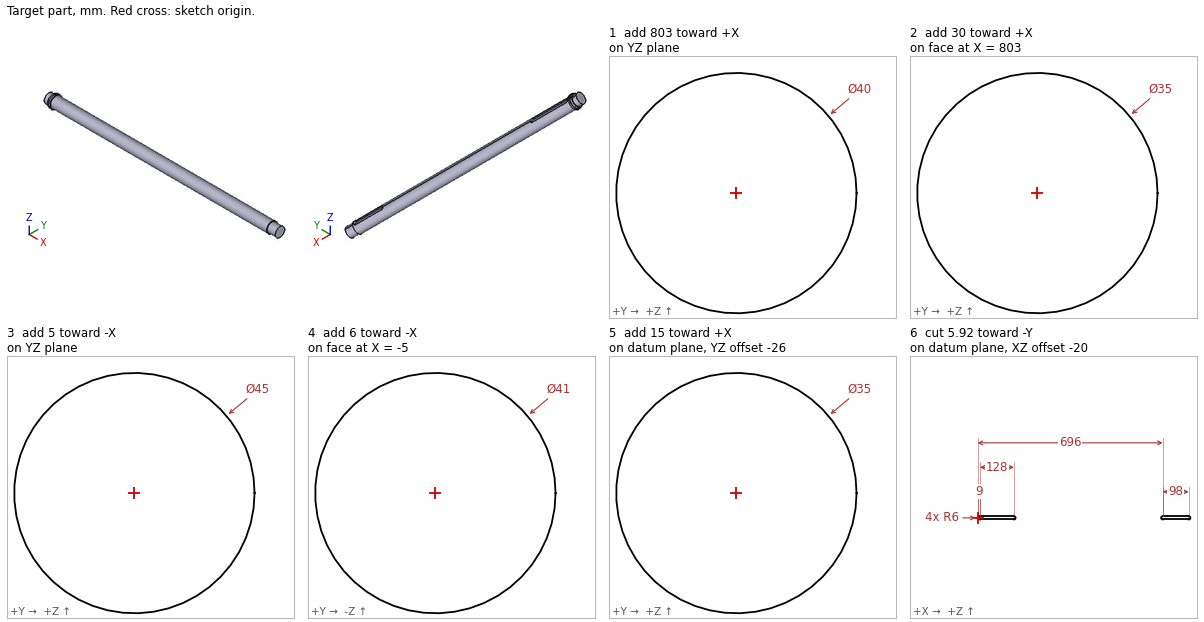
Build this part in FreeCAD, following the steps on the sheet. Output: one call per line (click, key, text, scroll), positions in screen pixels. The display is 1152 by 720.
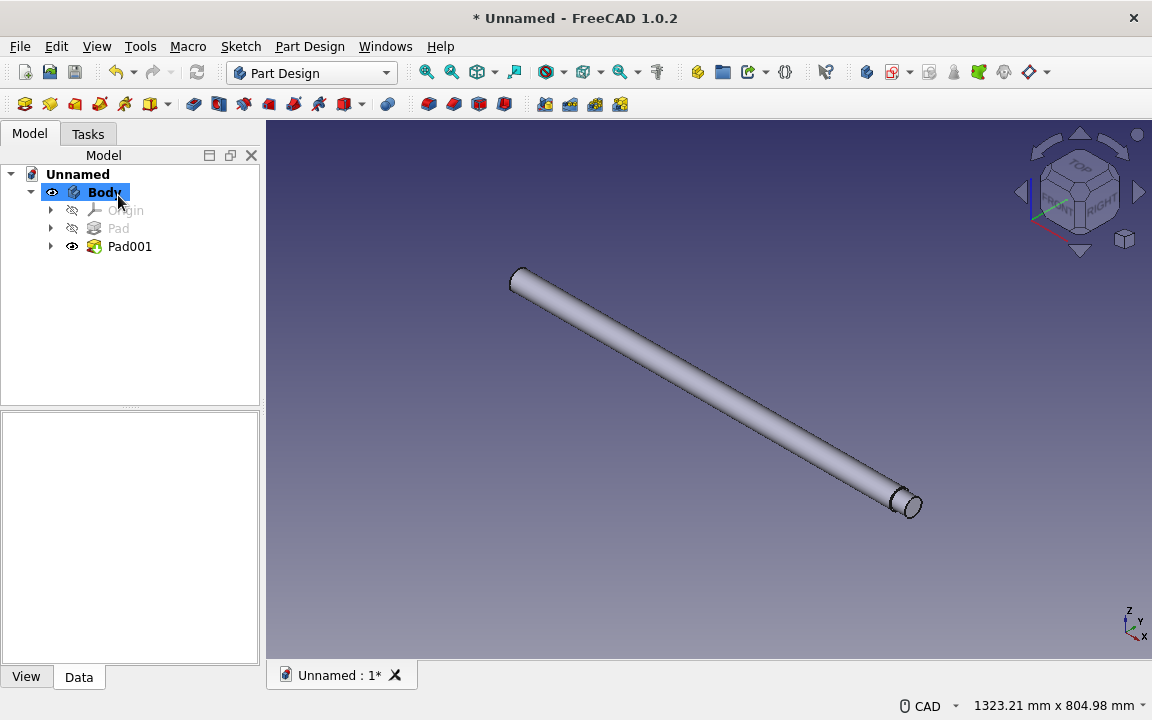
click(892, 72)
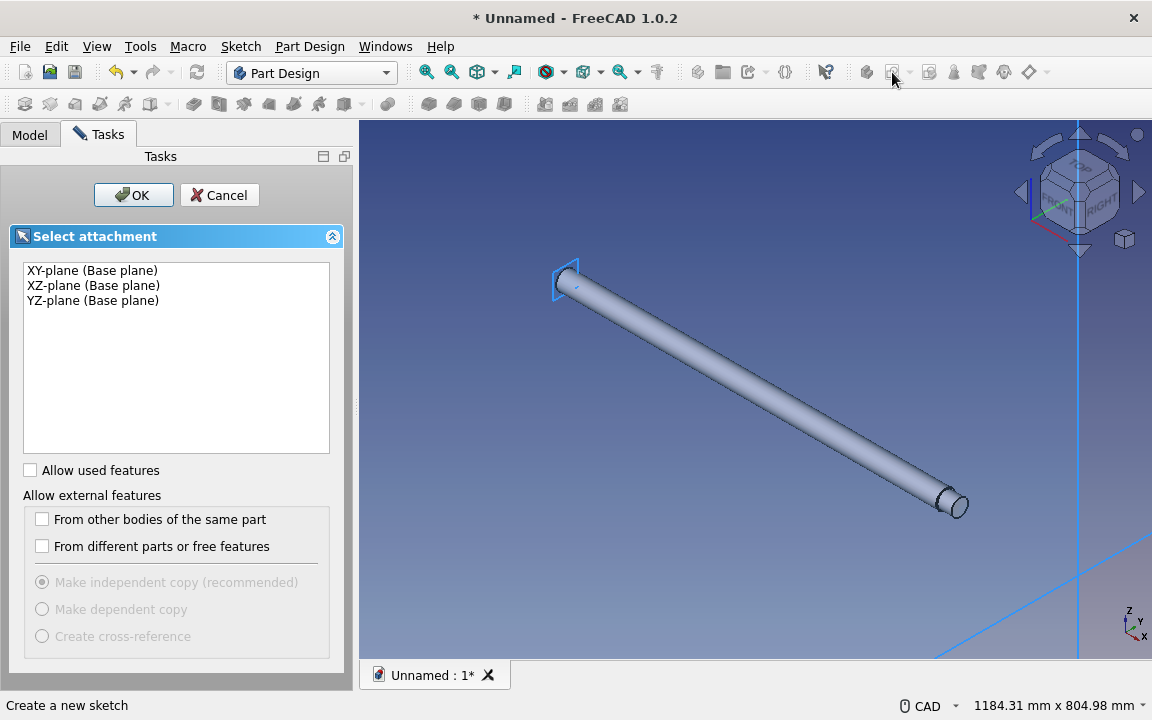
click(84, 300)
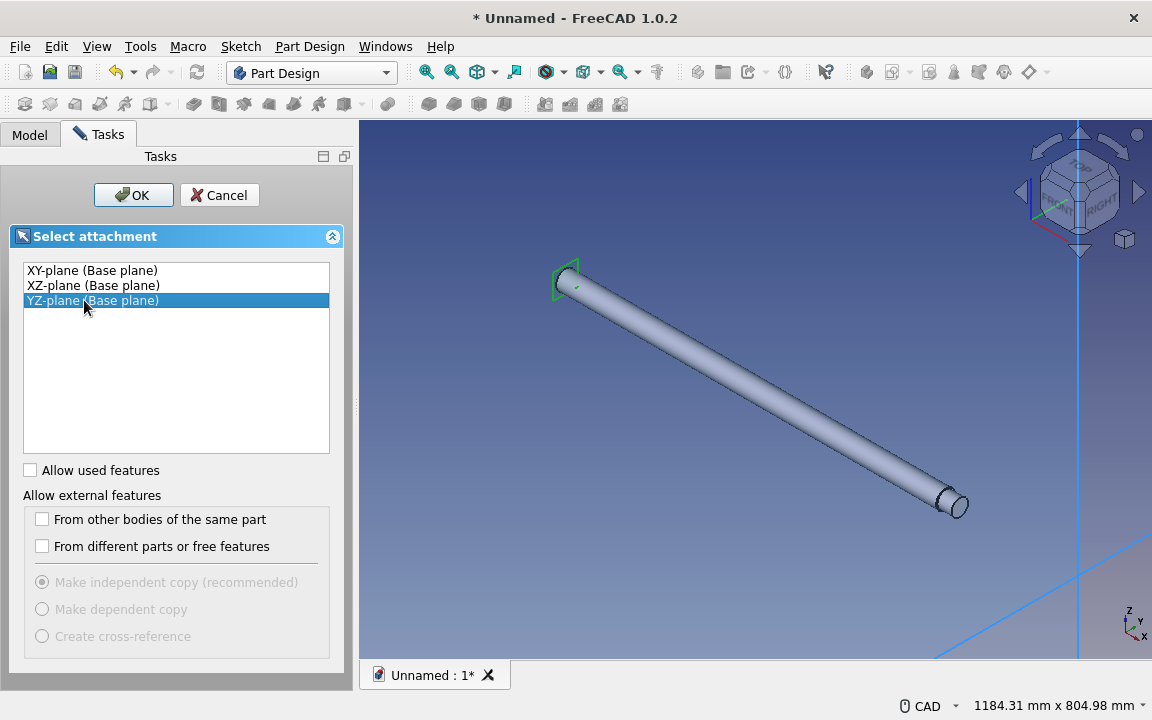
click(134, 195)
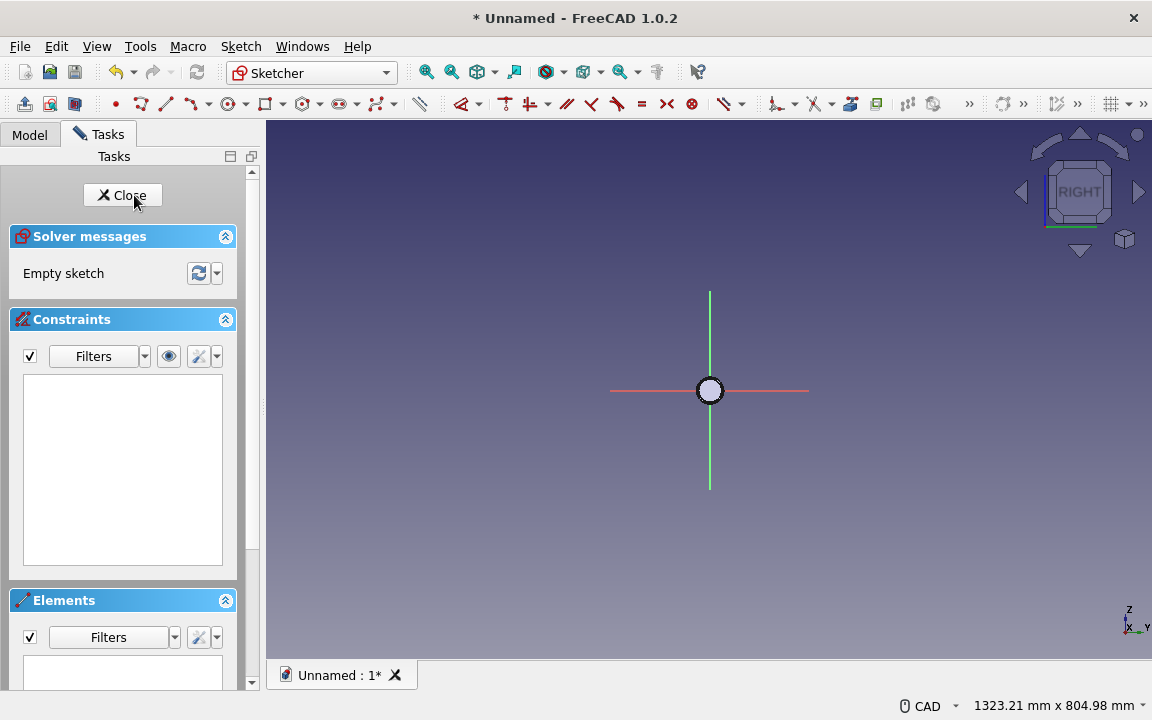
click(75, 104)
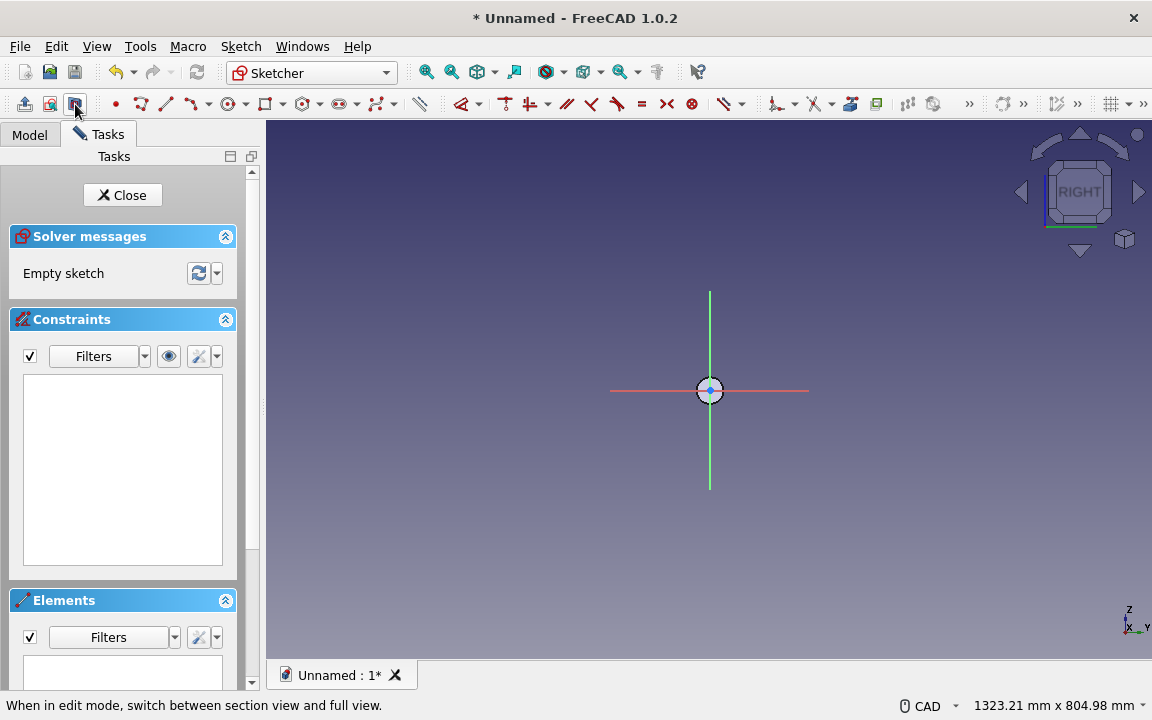
scroll(717, 391, up, 12)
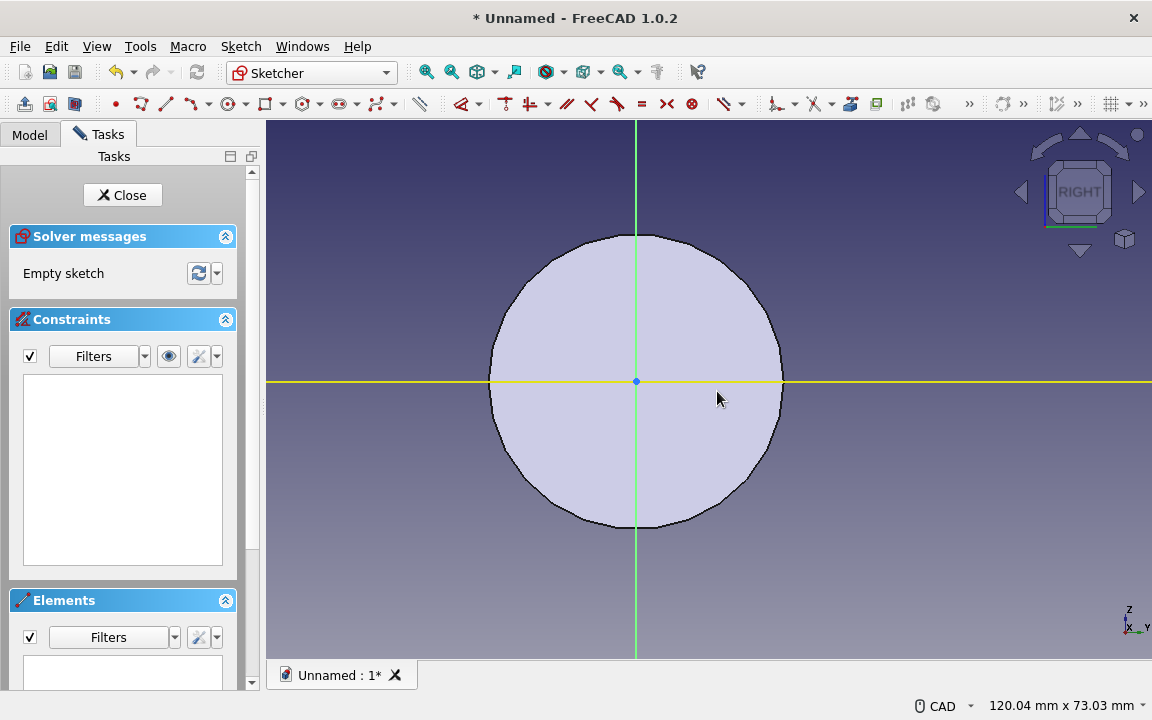
click(228, 104)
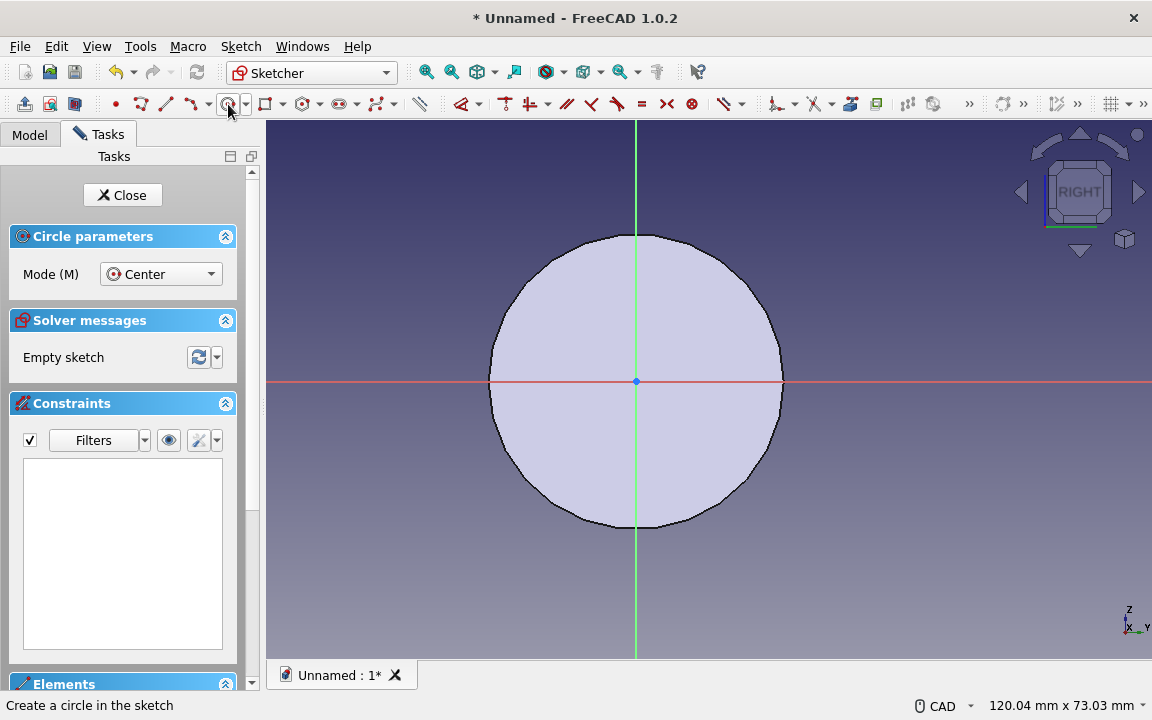
click(636, 382)
move(754, 264)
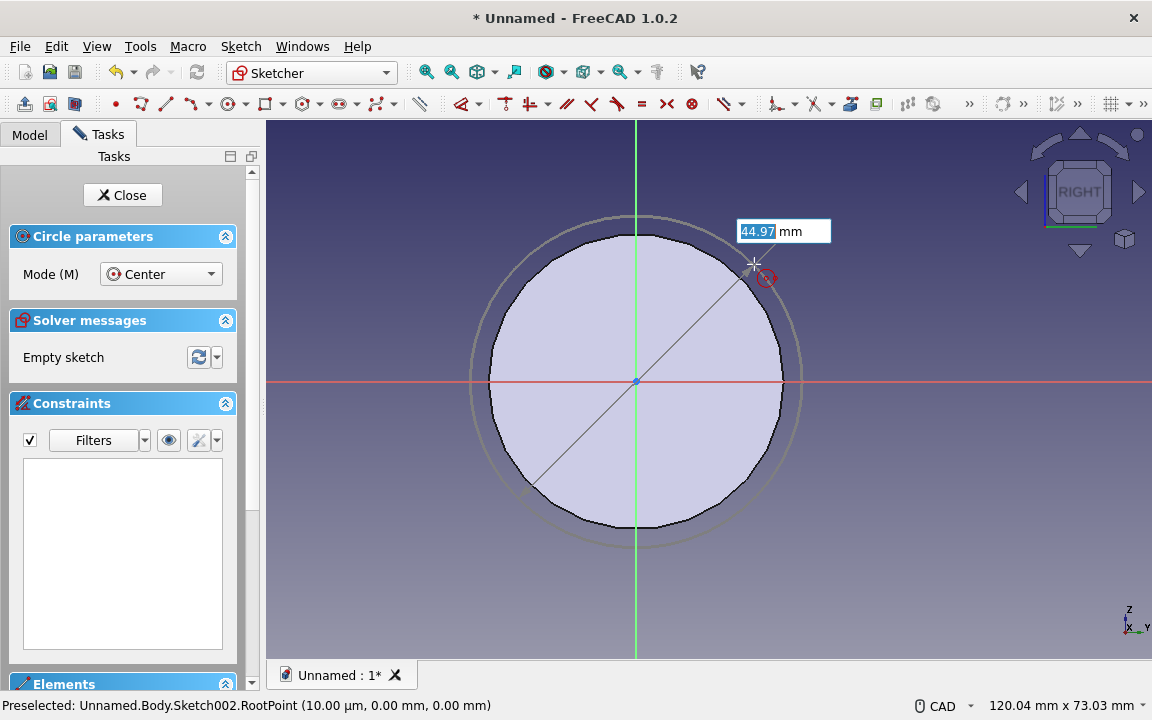
text(45)
key(Return)
key(Escape)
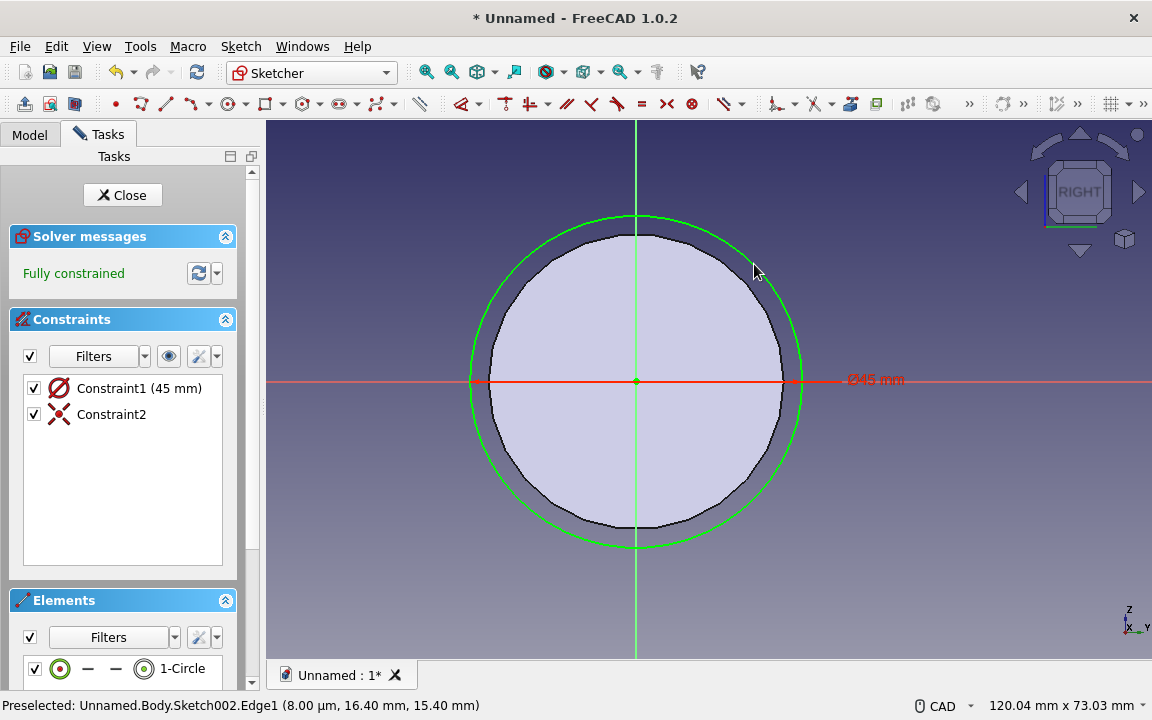
click(123, 195)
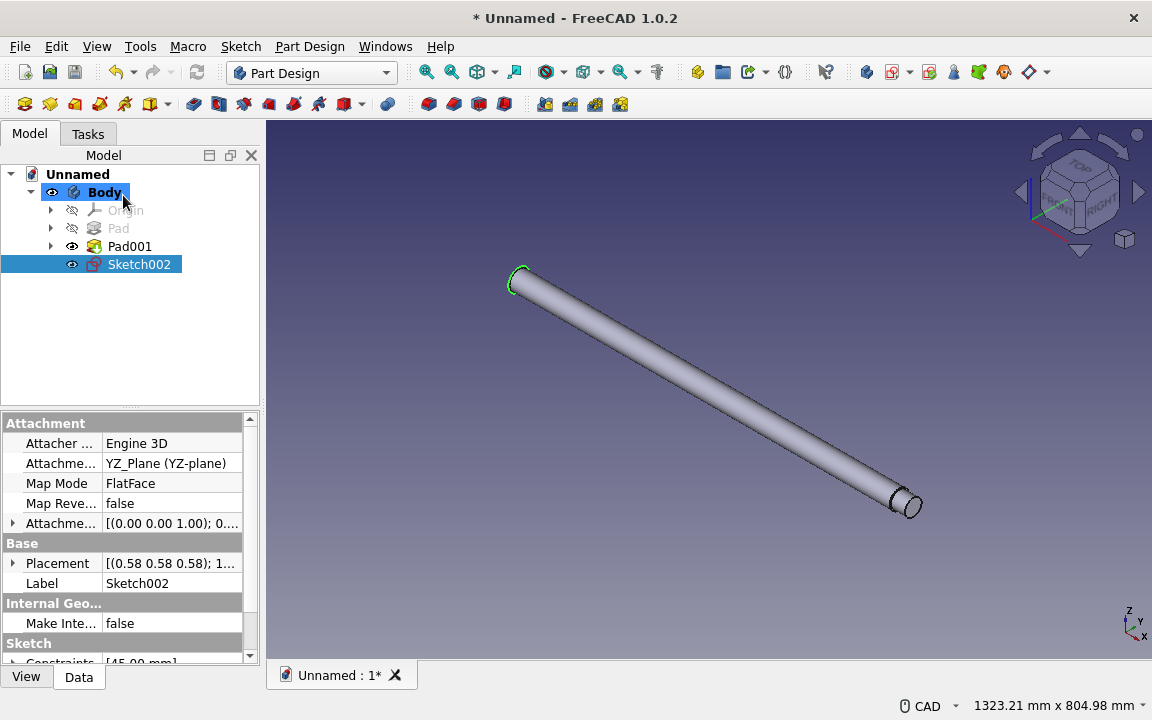
click(25, 104)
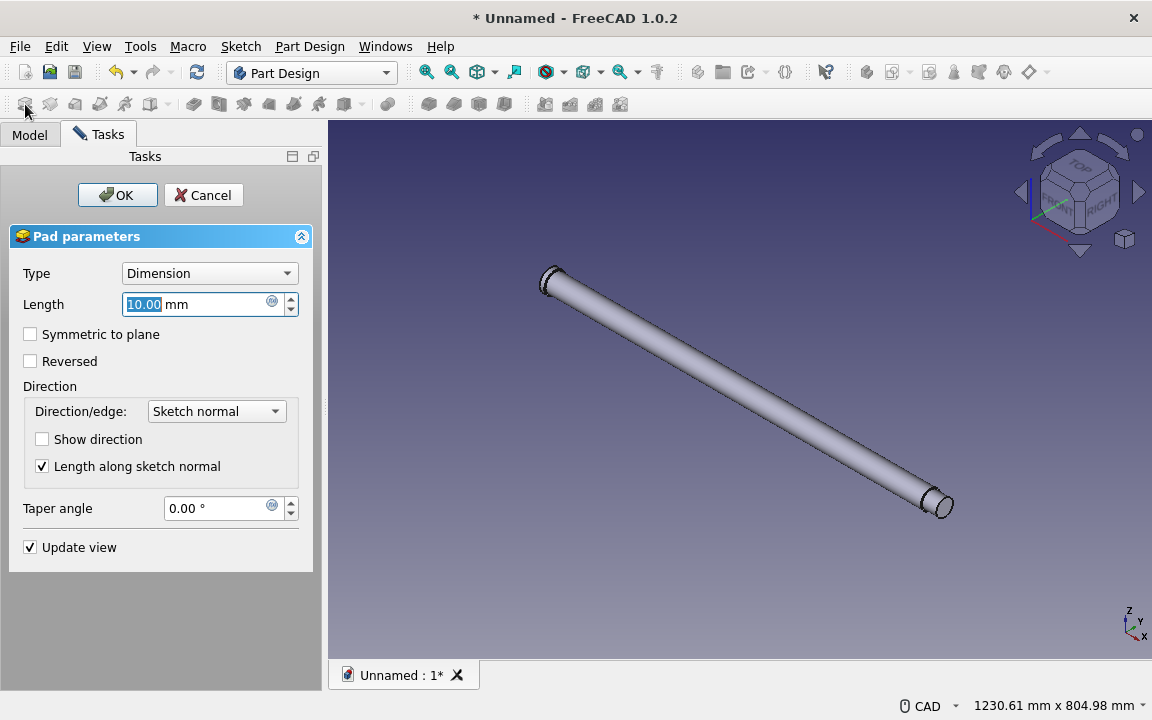
text(5)
key(Tab)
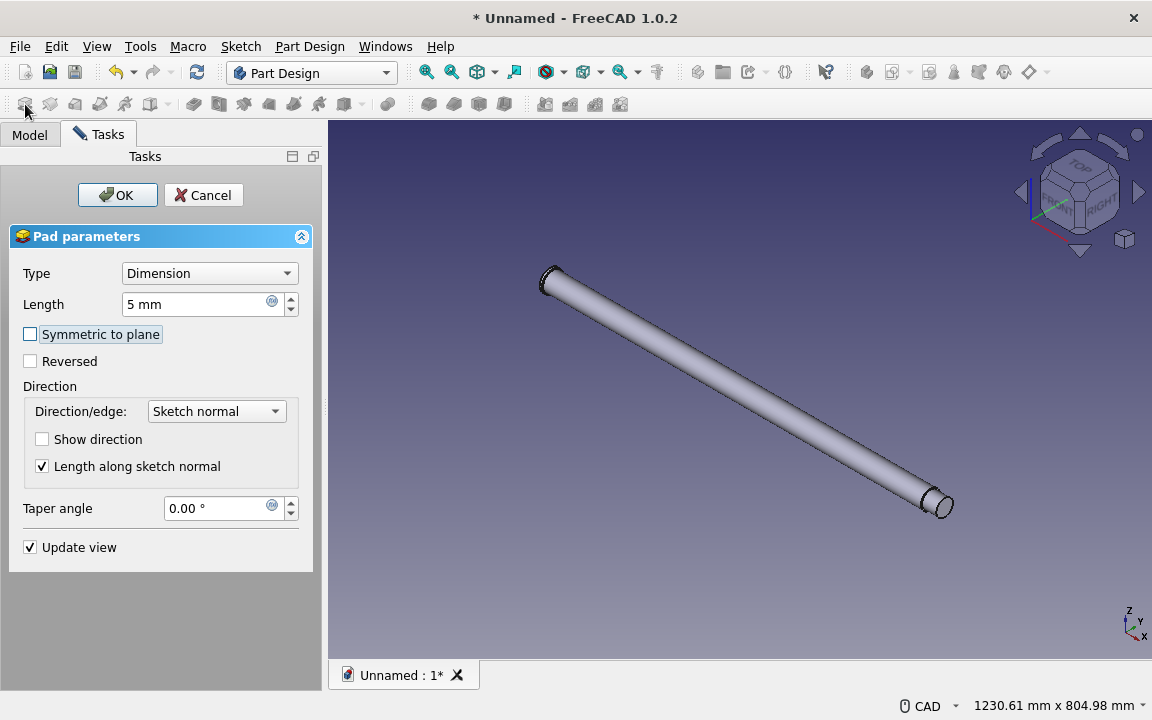
click(31, 361)